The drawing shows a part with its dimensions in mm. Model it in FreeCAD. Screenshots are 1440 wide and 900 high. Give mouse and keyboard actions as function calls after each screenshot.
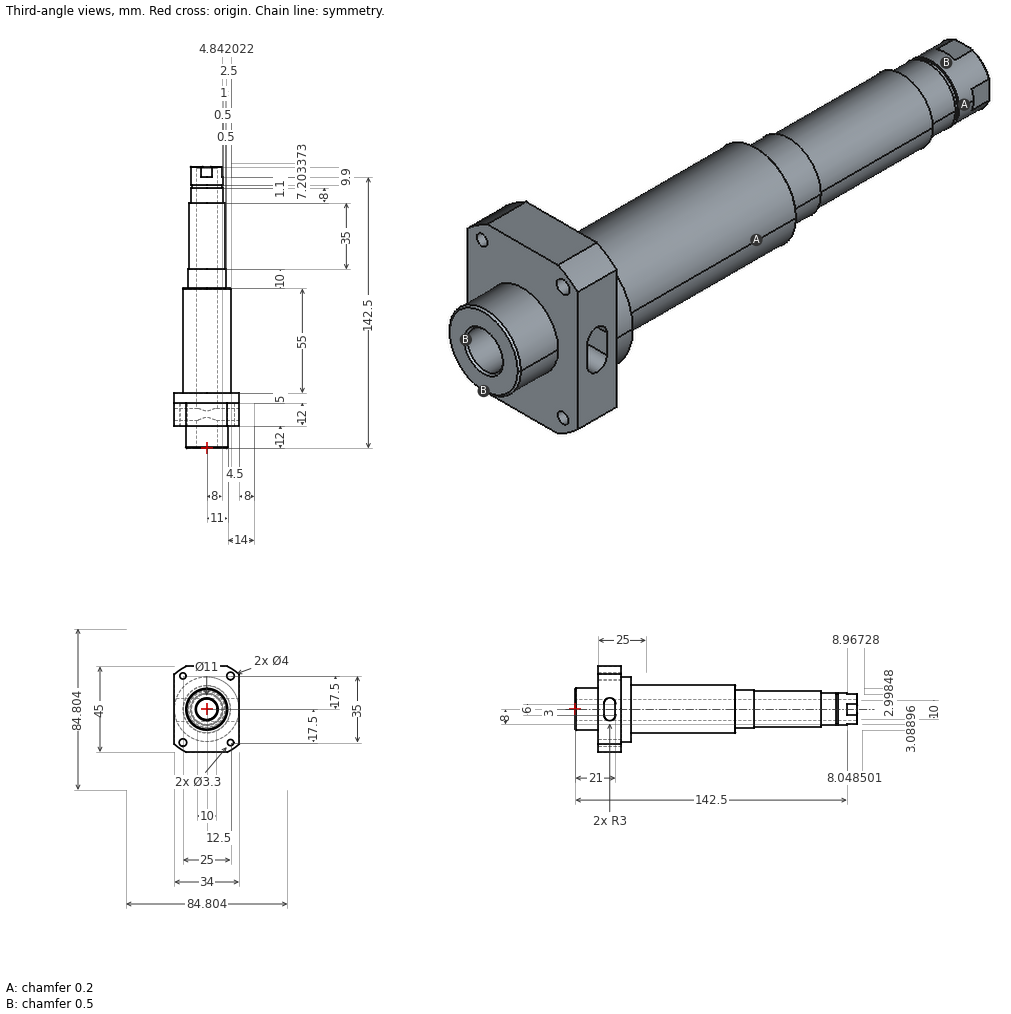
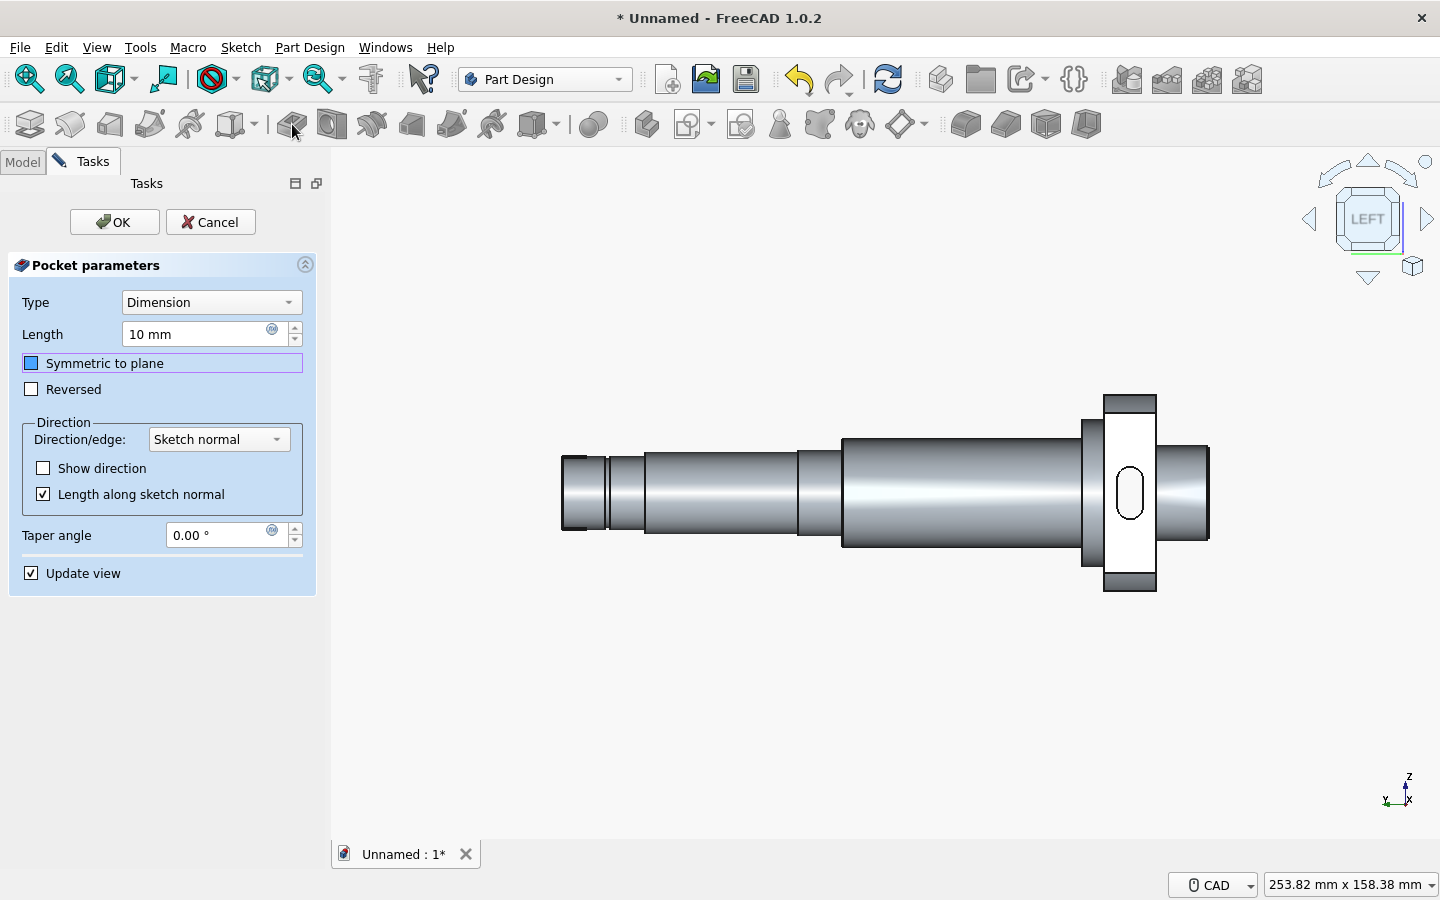
click(30, 363)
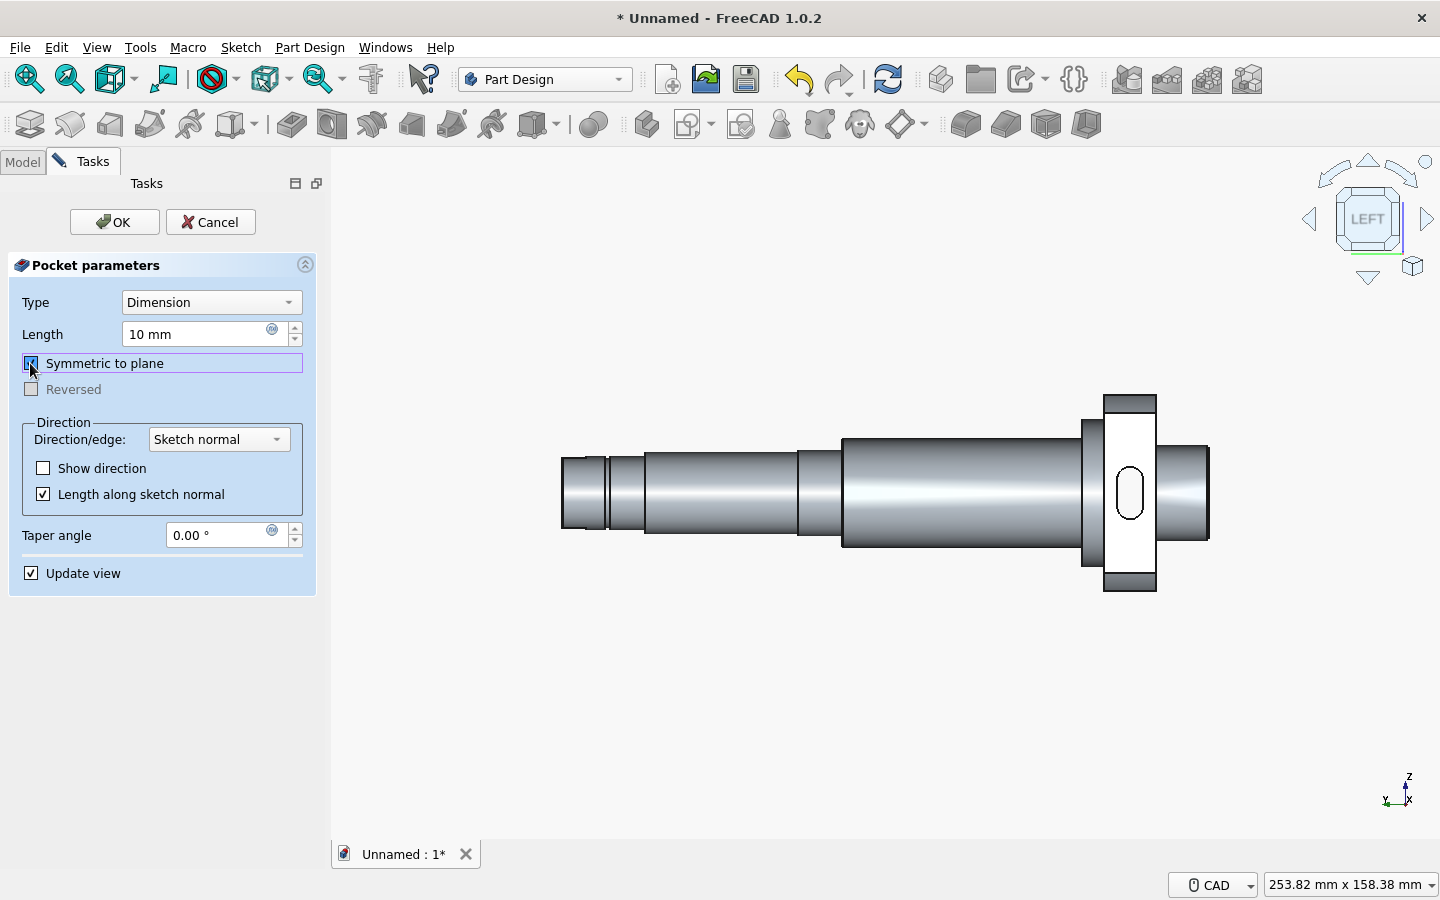
click(115, 222)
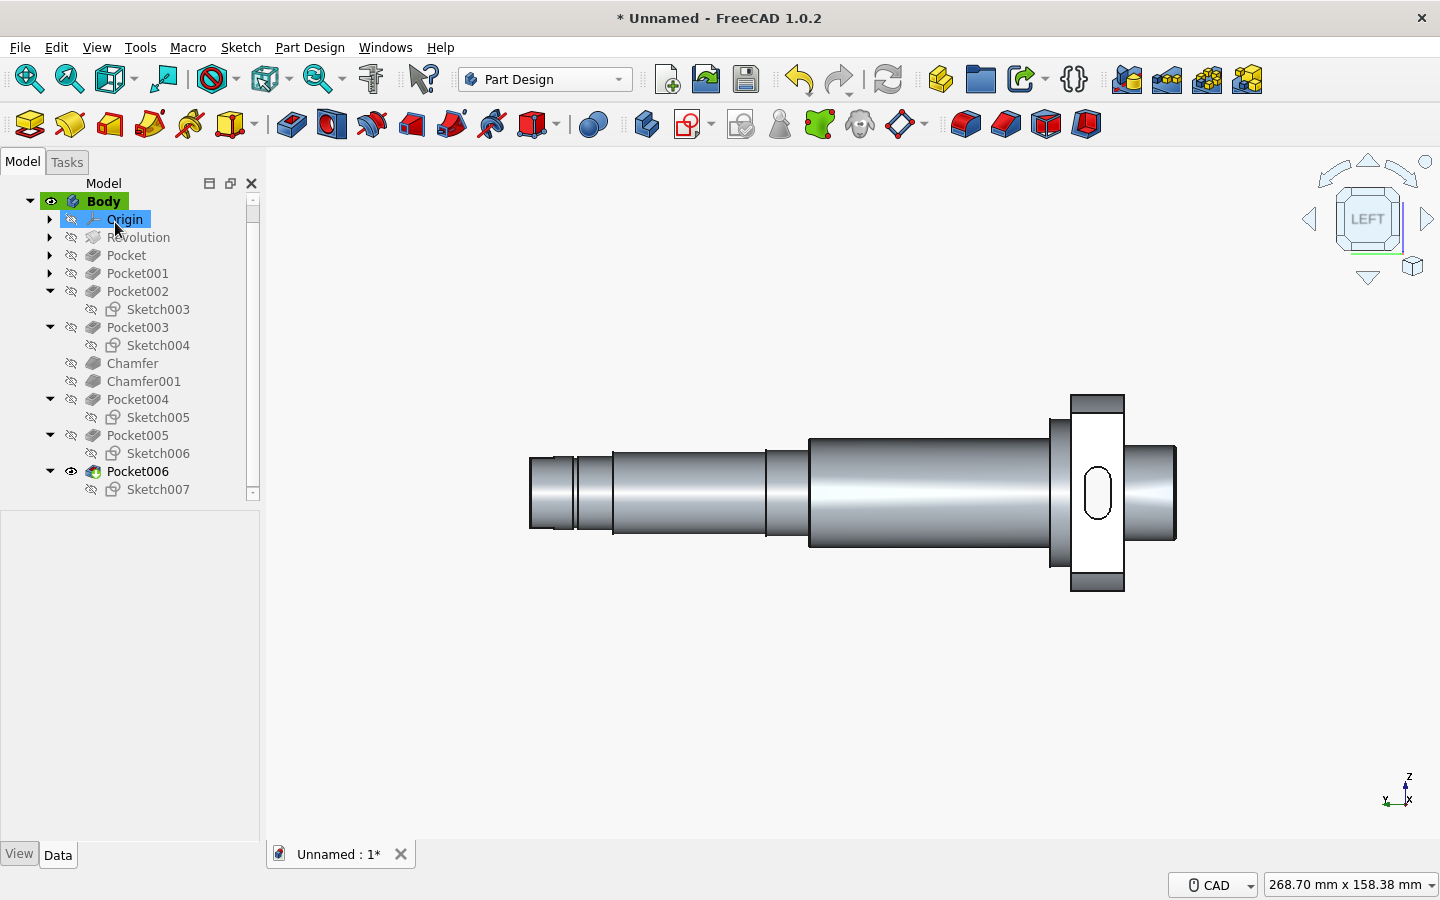
key(0)